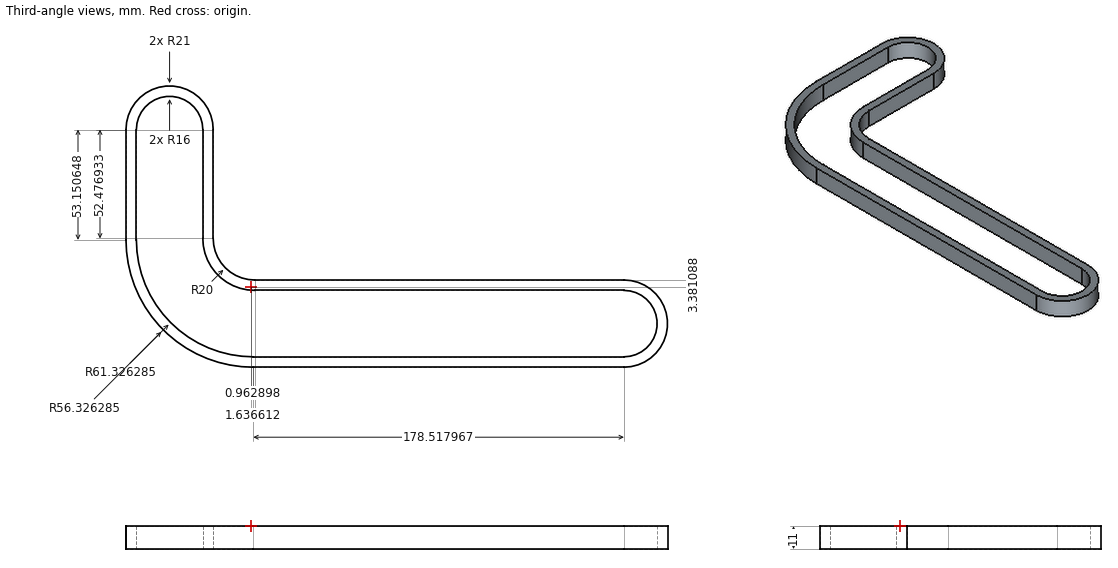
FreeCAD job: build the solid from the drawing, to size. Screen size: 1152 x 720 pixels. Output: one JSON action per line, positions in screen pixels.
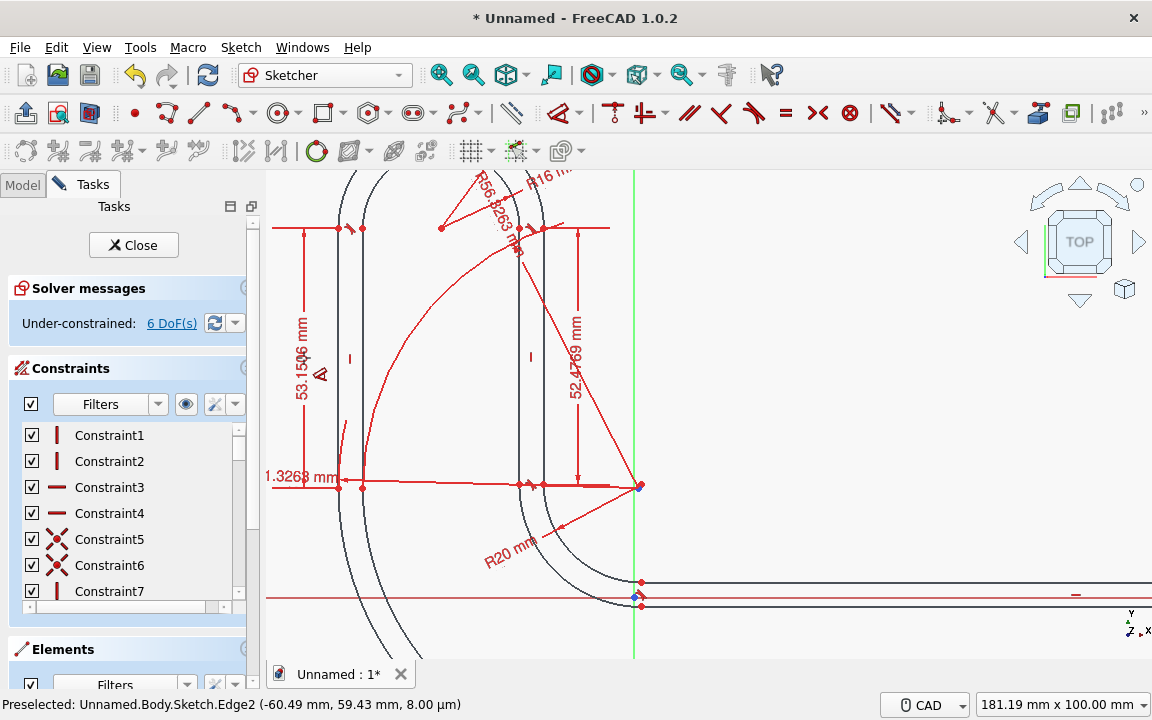
{"action": "left_click", "coordinate": [363, 410]}
{"action": "left_click", "coordinate": [397, 358]}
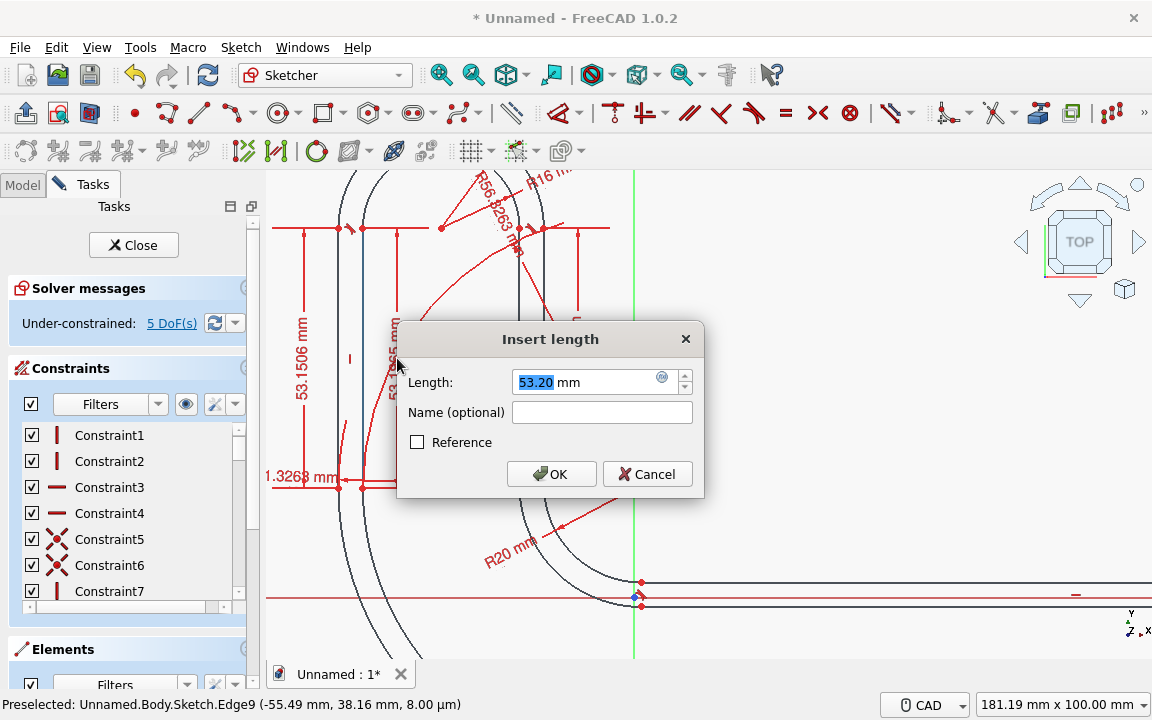
{"action": "type", "text": "53.150648"}
{"action": "key", "text": "Return"}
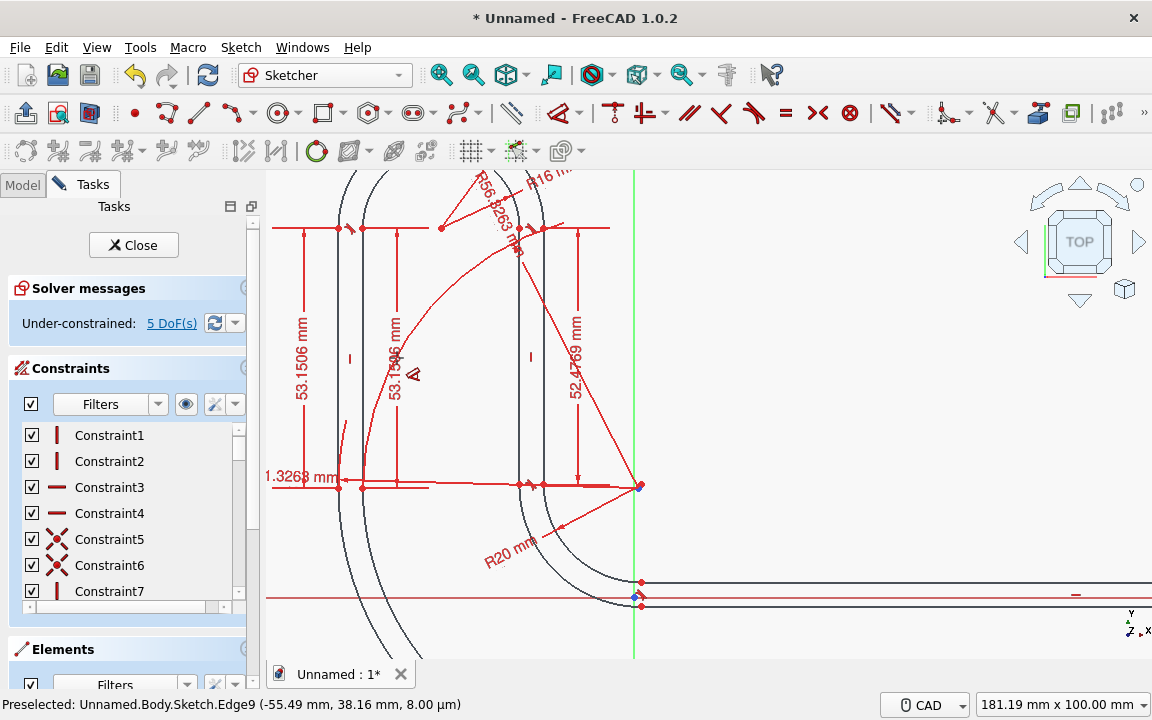
{"action": "scroll", "coordinate": [445, 391], "scroll_direction": "down", "scroll_amount": 5}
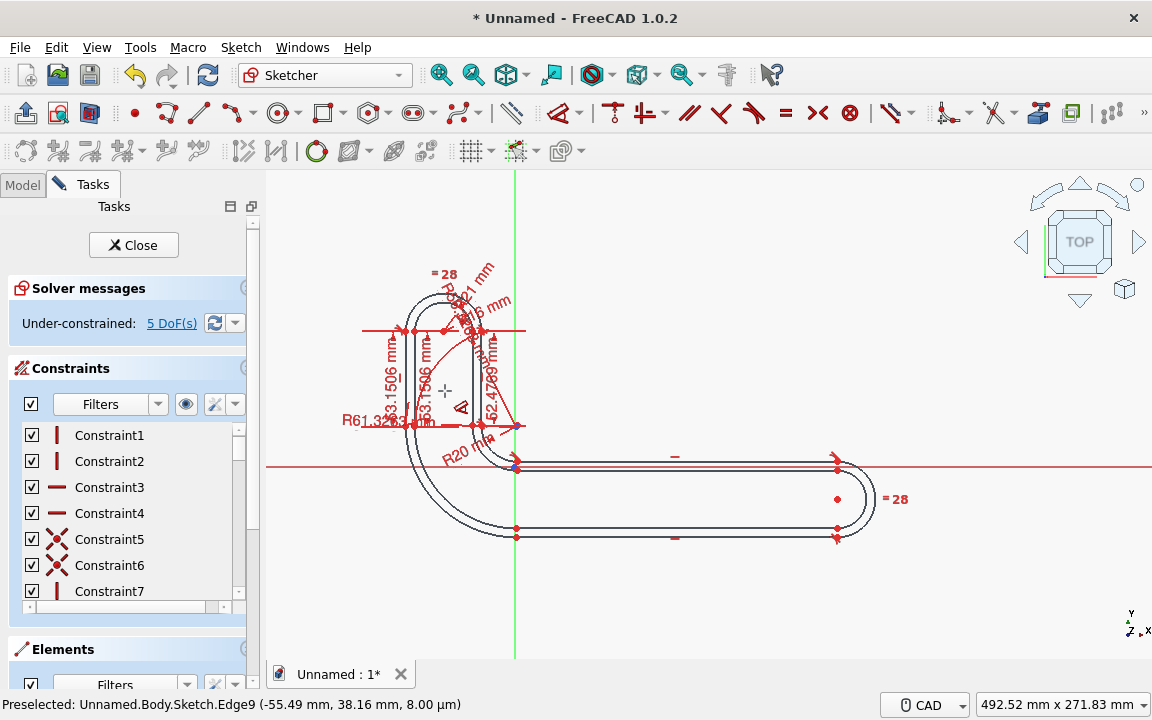
{"action": "scroll", "coordinate": [517, 537], "scroll_direction": "up", "scroll_amount": 16}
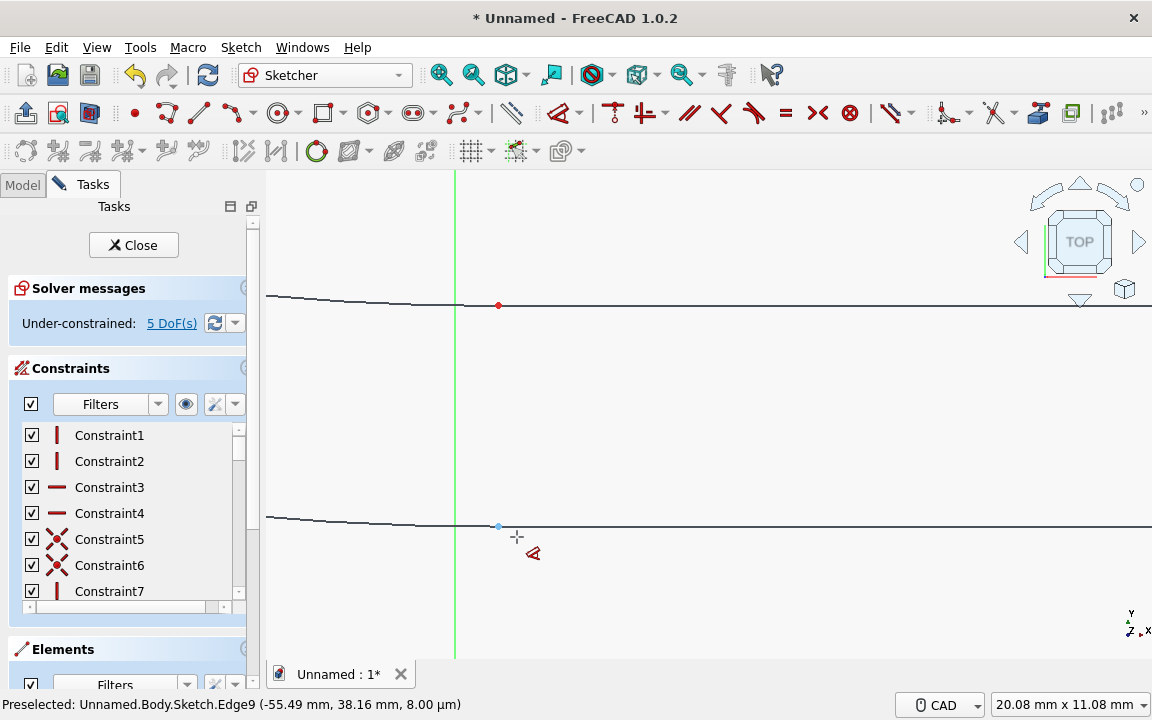
{"action": "left_click", "coordinate": [499, 527]}
{"action": "left_click", "coordinate": [477, 561]}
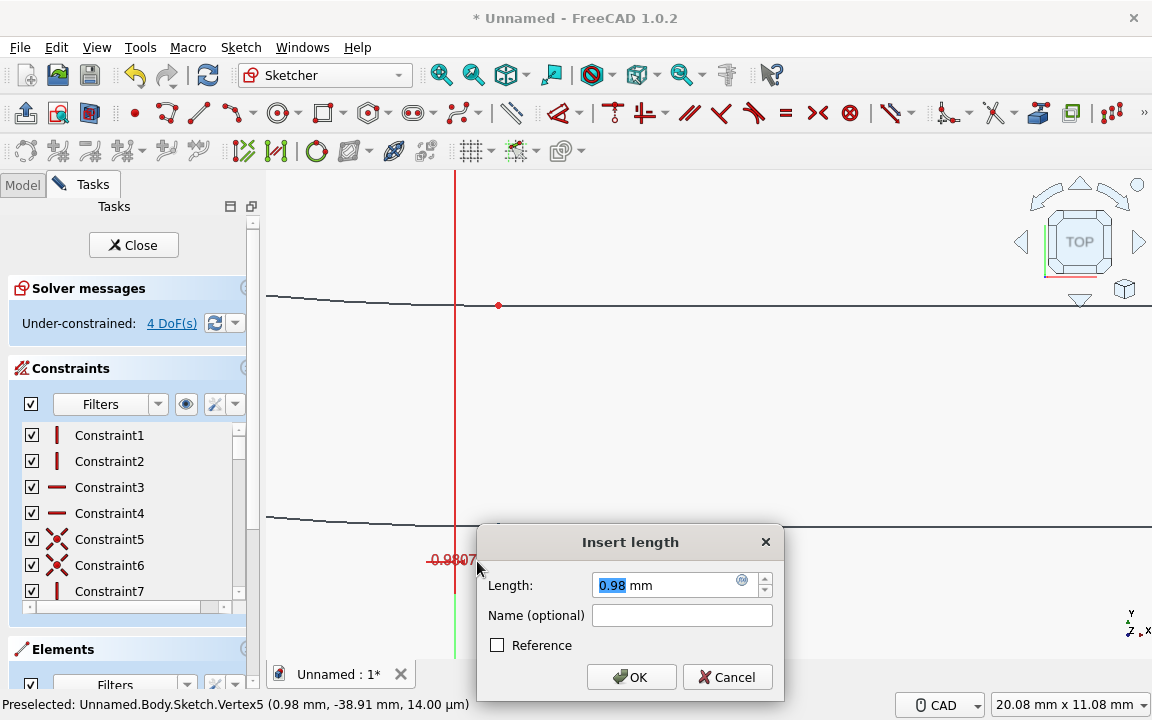
{"action": "type", "text": "0.962898"}
{"action": "key", "text": "Return"}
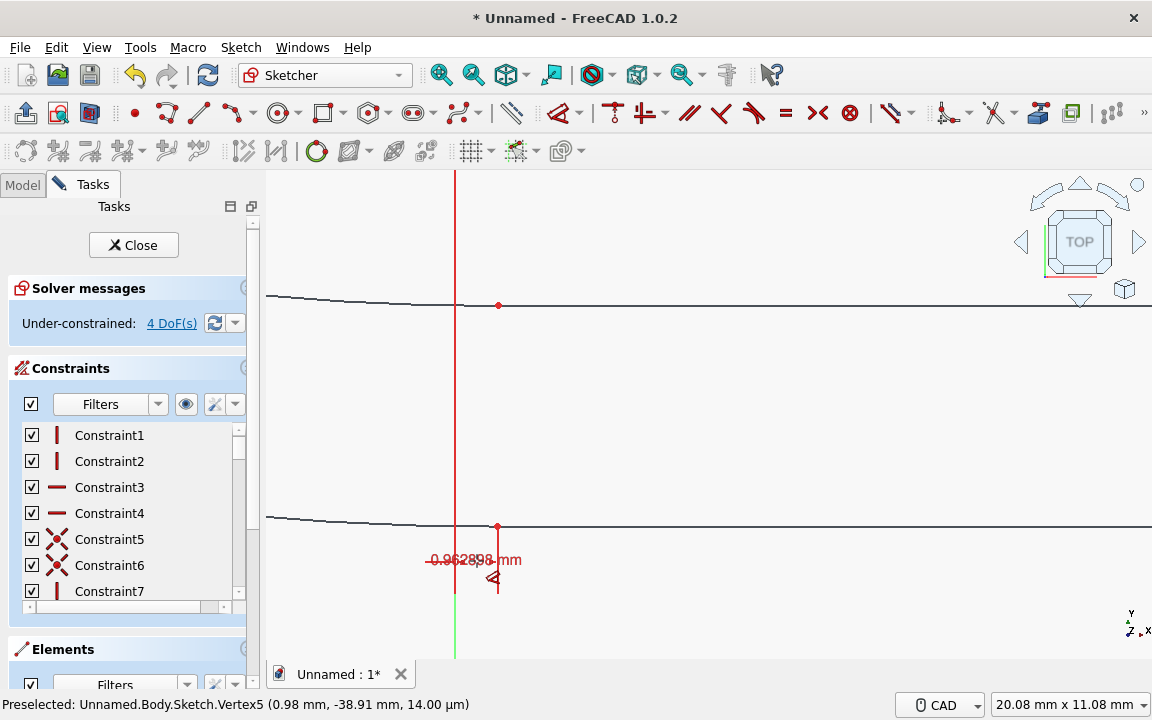
{"action": "scroll", "coordinate": [488, 566], "scroll_direction": "down", "scroll_amount": 15}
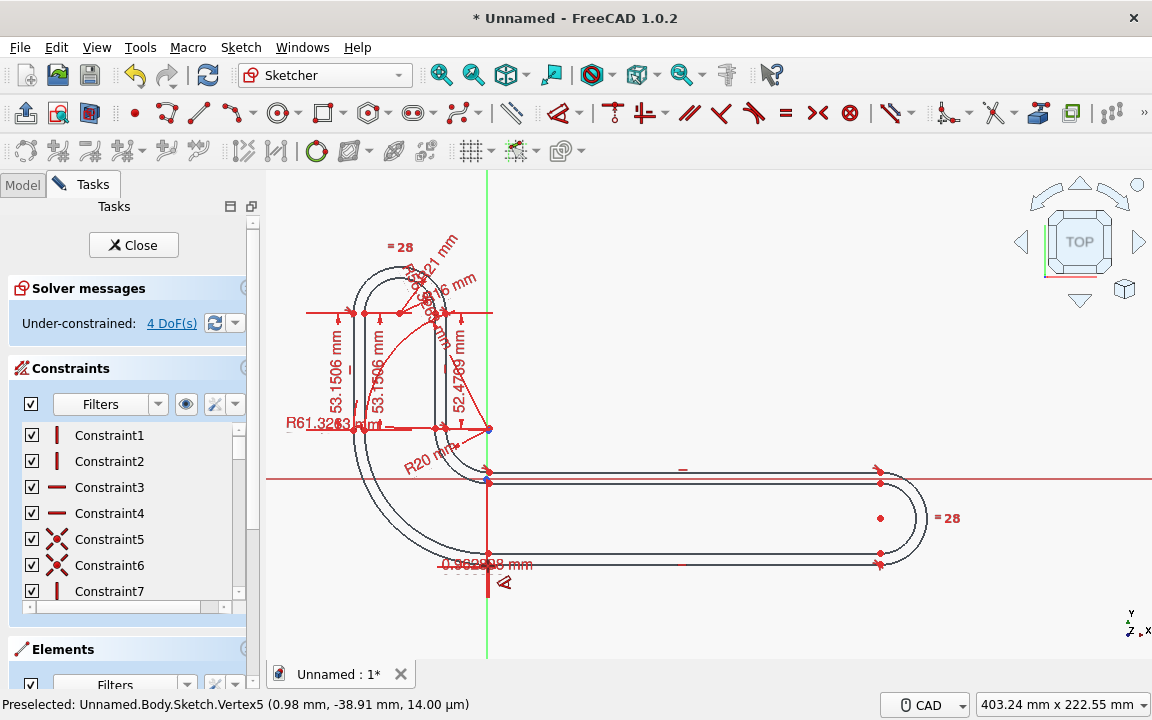
{"action": "scroll", "coordinate": [881, 473], "scroll_direction": "up", "scroll_amount": 9}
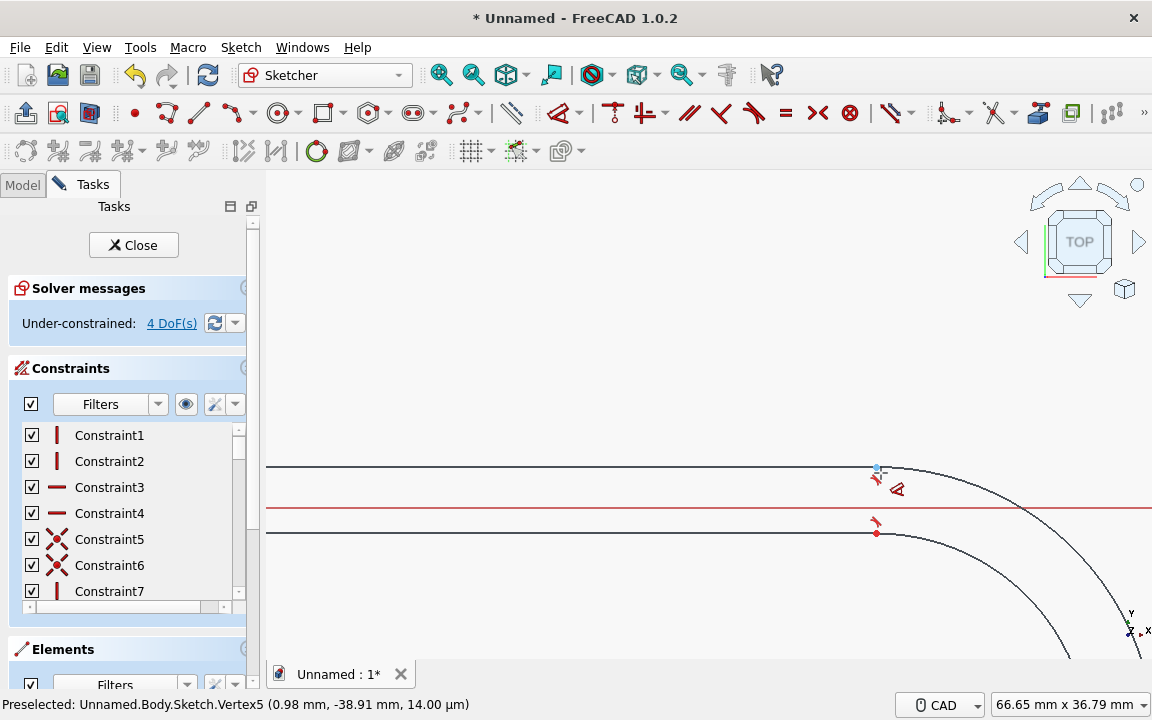
{"action": "left_click", "coordinate": [876, 467]}
{"action": "left_click", "coordinate": [910, 488]}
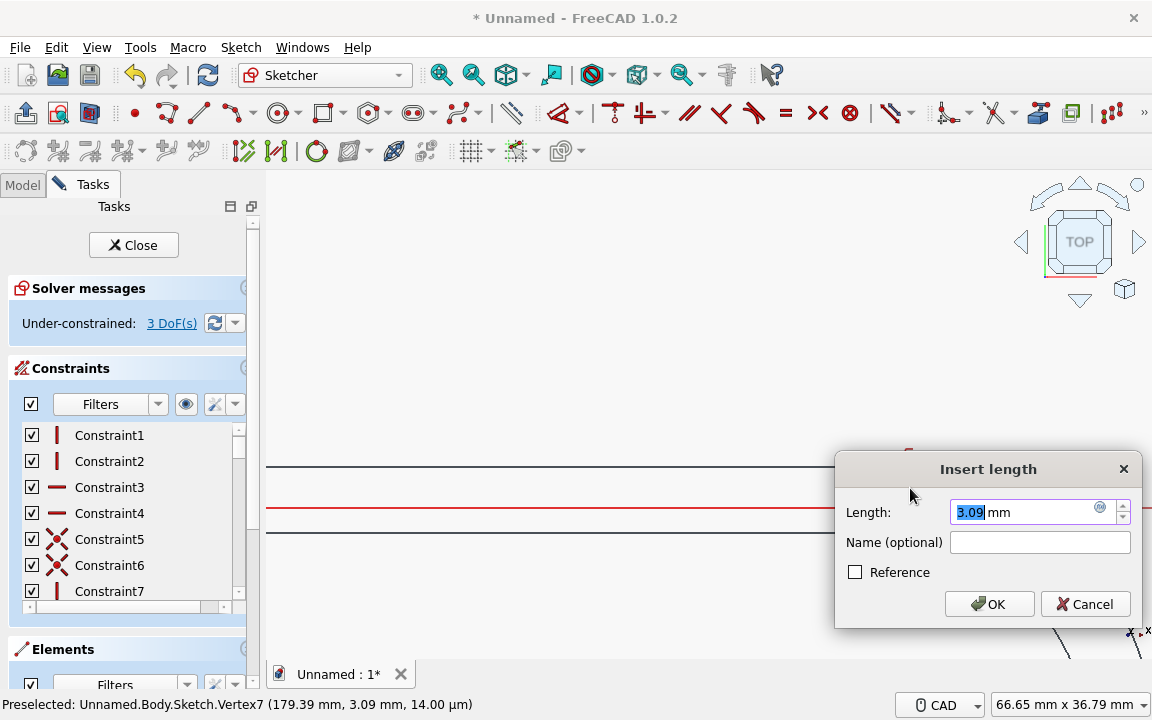
{"action": "type", "text": "3.381088"}
{"action": "key", "text": "Return"}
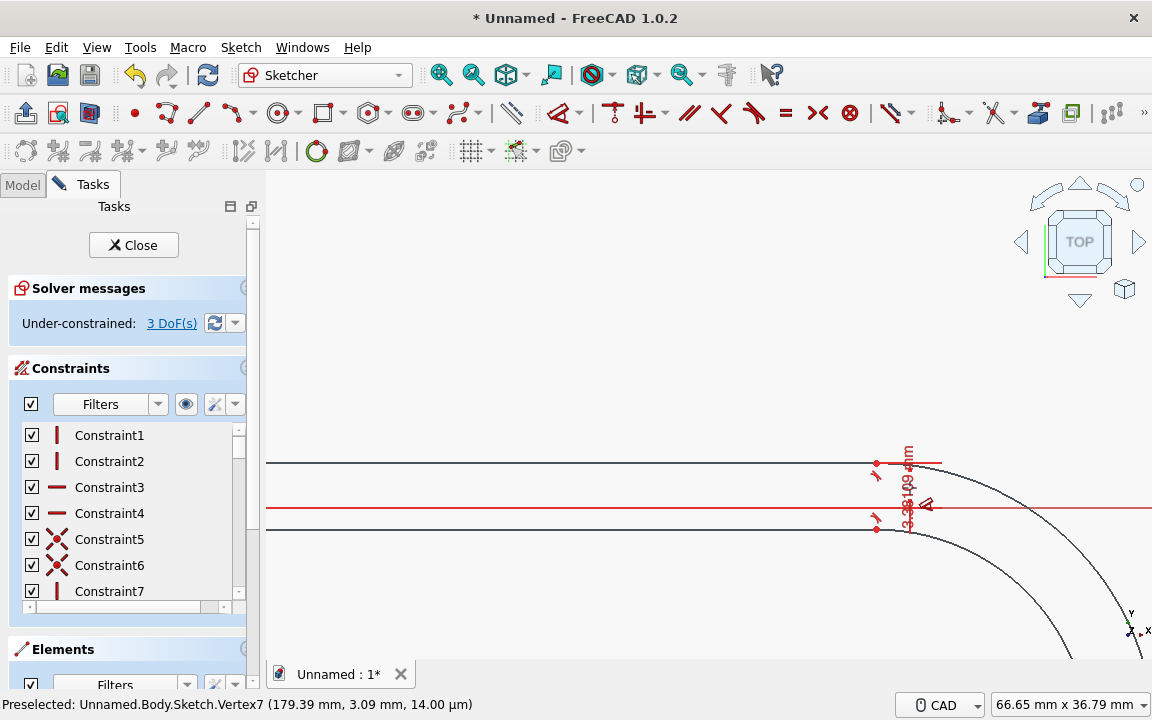
{"action": "scroll", "coordinate": [831, 460], "scroll_direction": "down", "scroll_amount": 10}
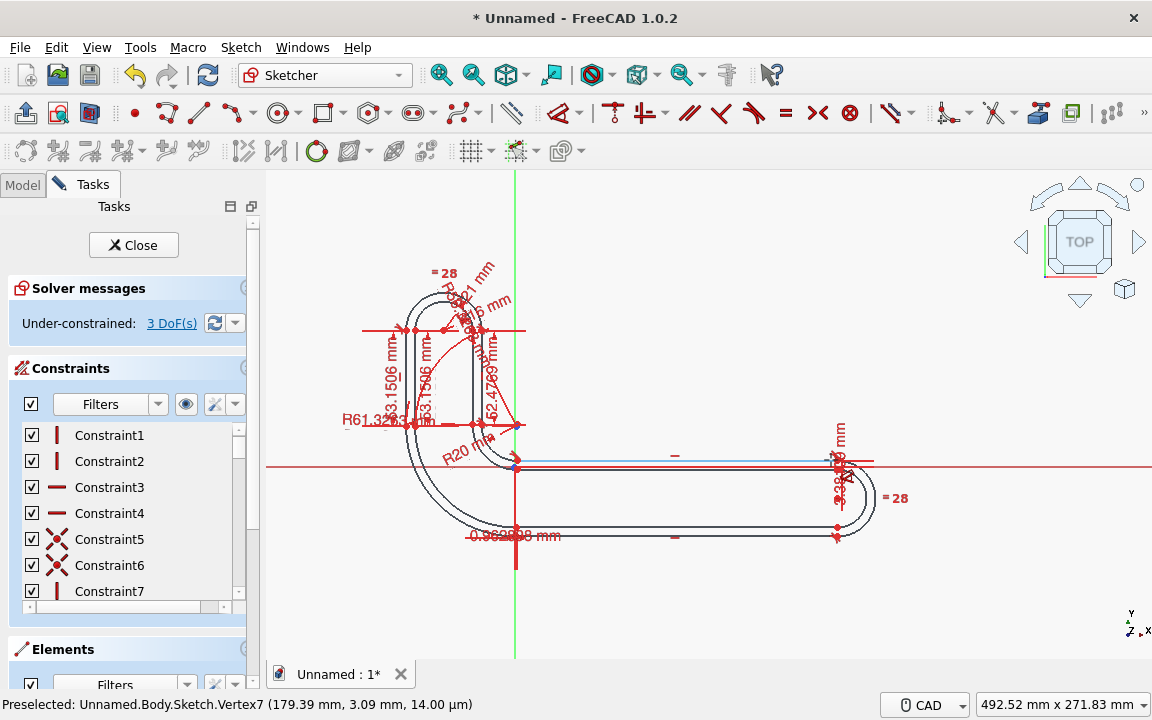
{"action": "scroll", "coordinate": [518, 461], "scroll_direction": "up", "scroll_amount": 14}